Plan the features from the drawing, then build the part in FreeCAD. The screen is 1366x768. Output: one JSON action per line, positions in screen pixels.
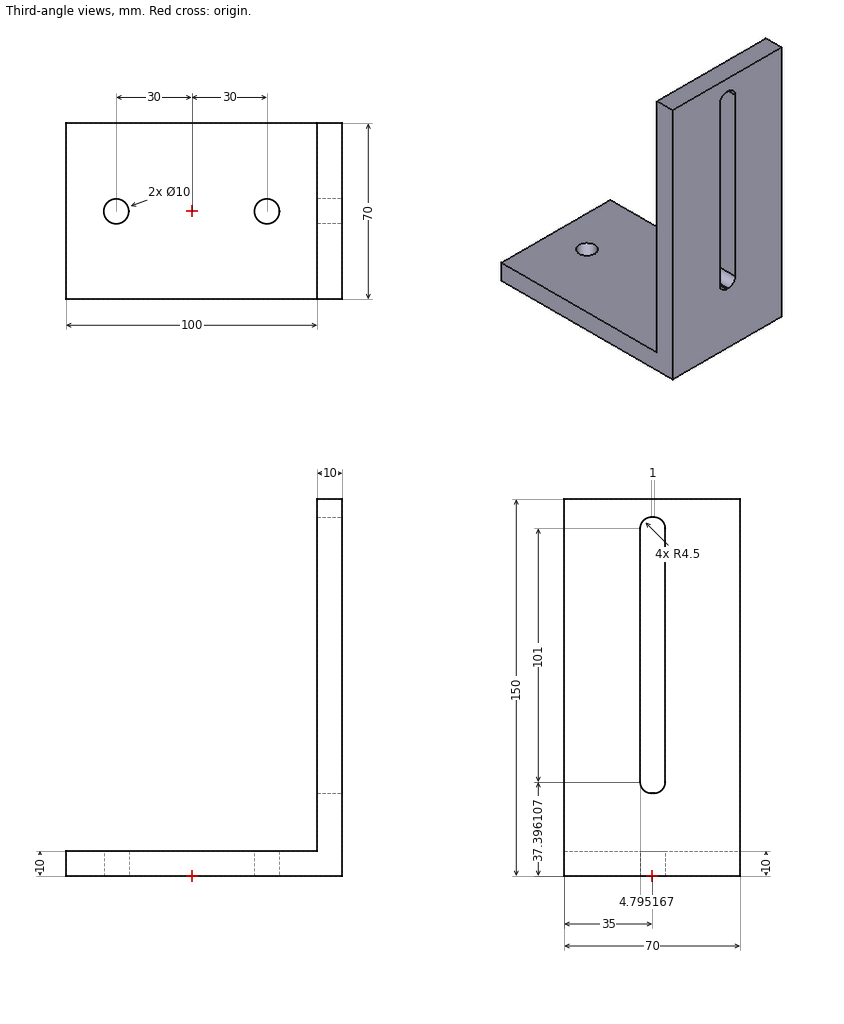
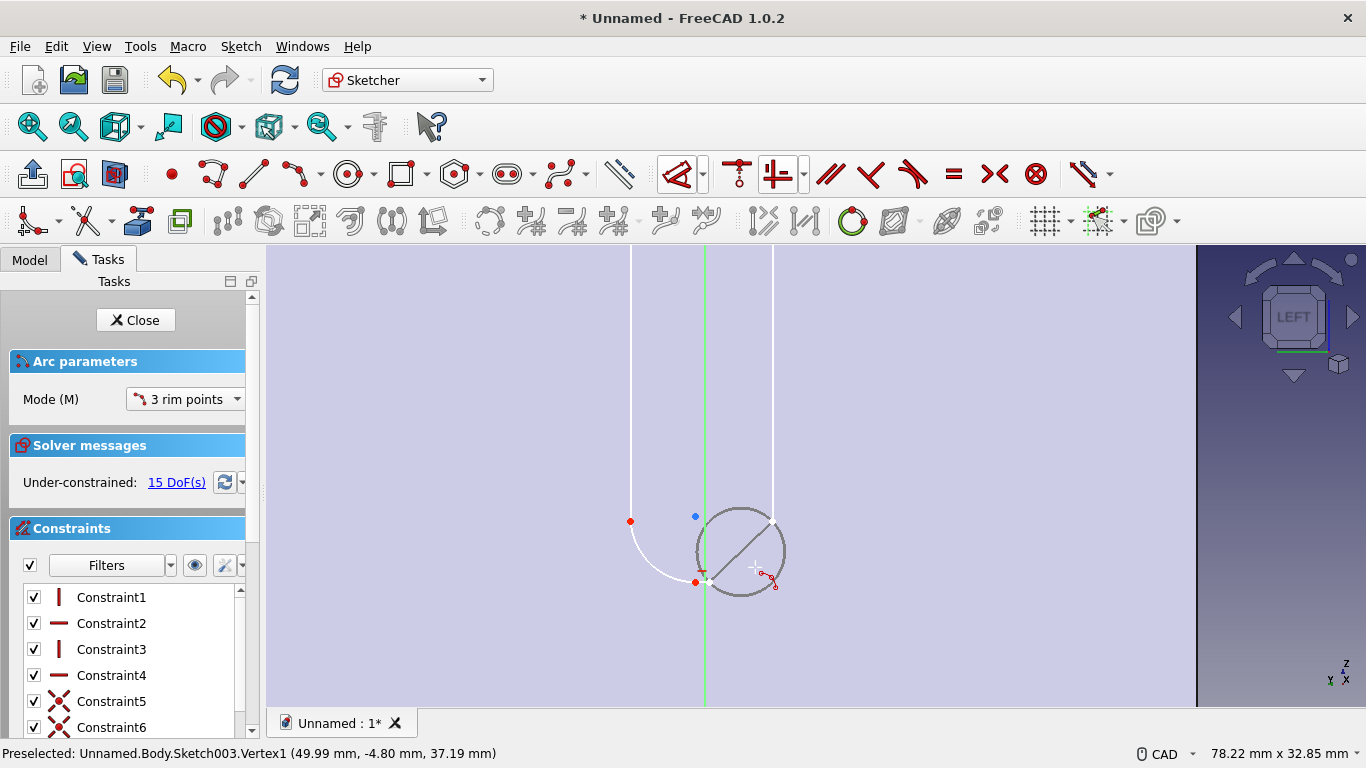
{"action": "left_click", "coordinate": [754, 563]}
{"action": "key", "text": "Escape"}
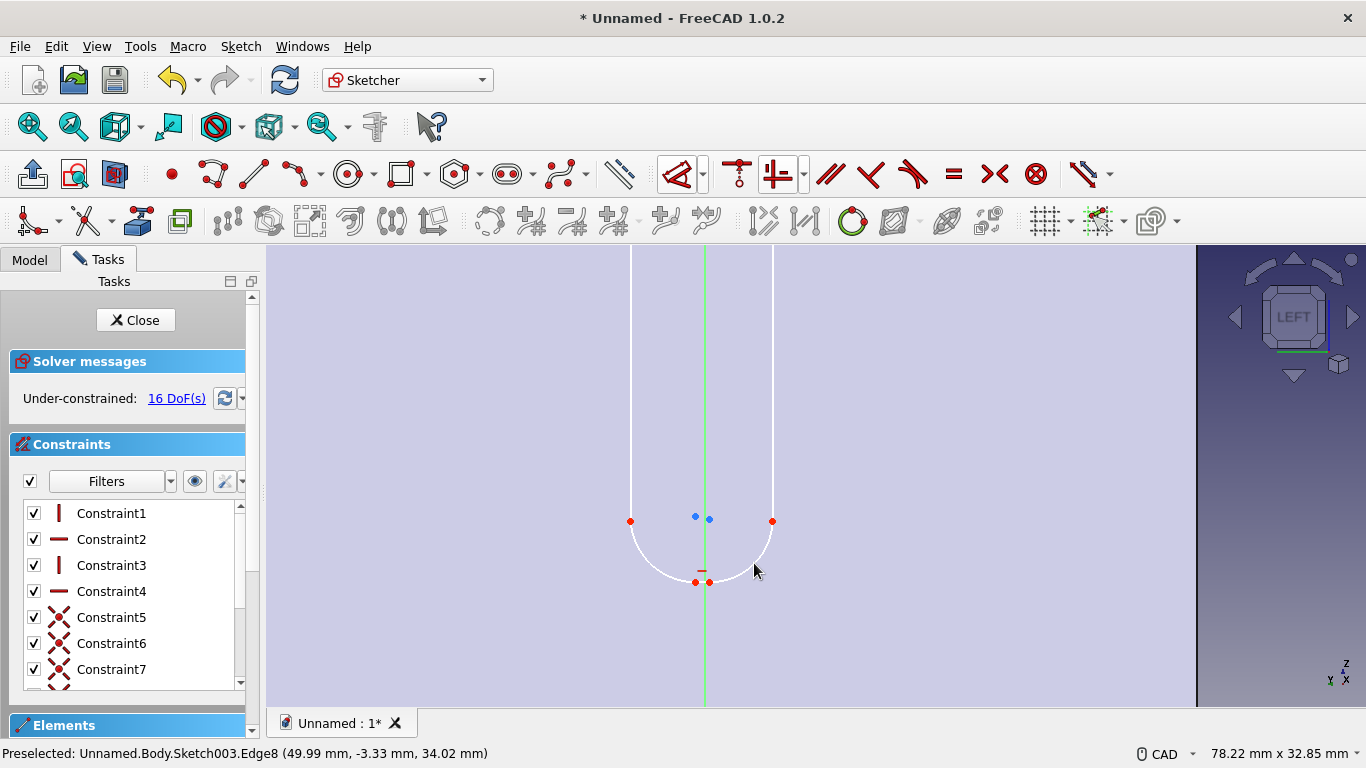
{"action": "scroll", "coordinate": [755, 544], "scroll_direction": "down", "scroll_amount": 10}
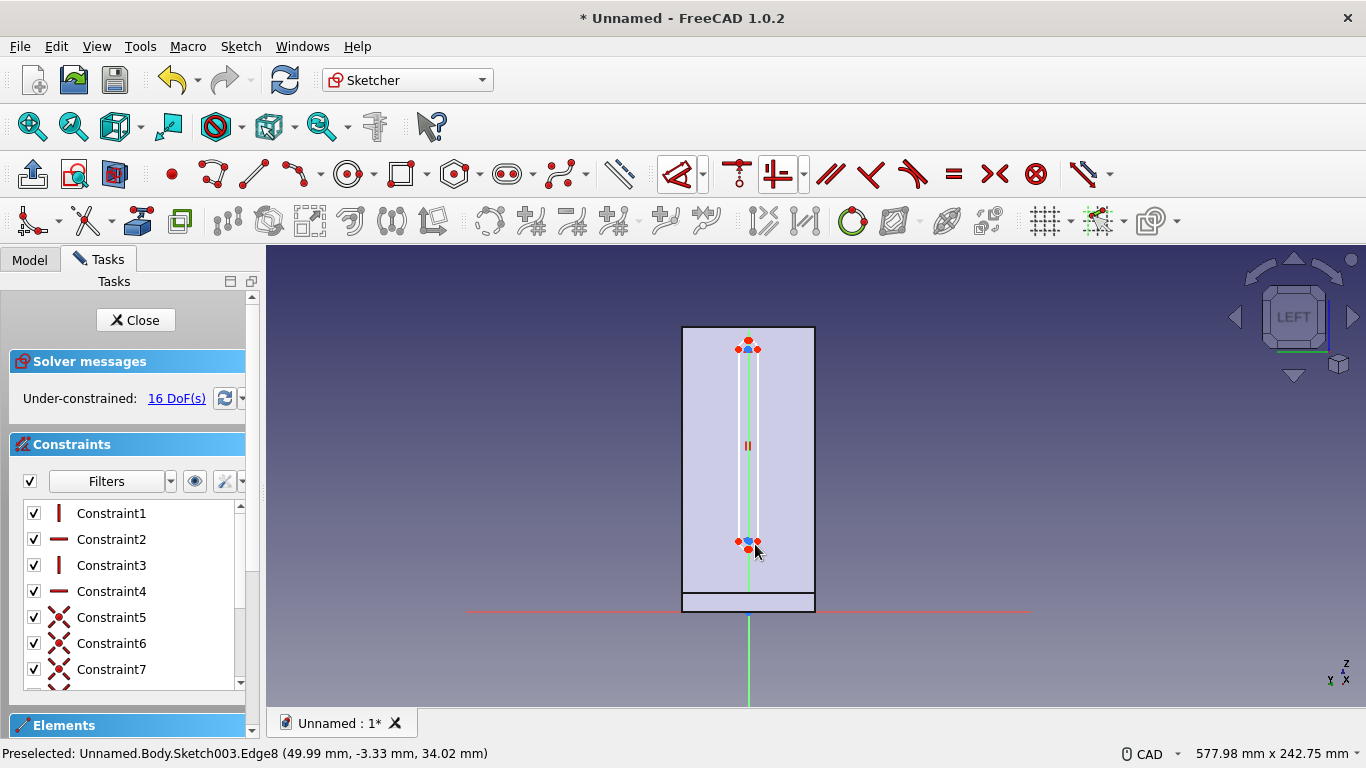
{"action": "scroll", "coordinate": [758, 484], "scroll_direction": "up", "scroll_amount": 3}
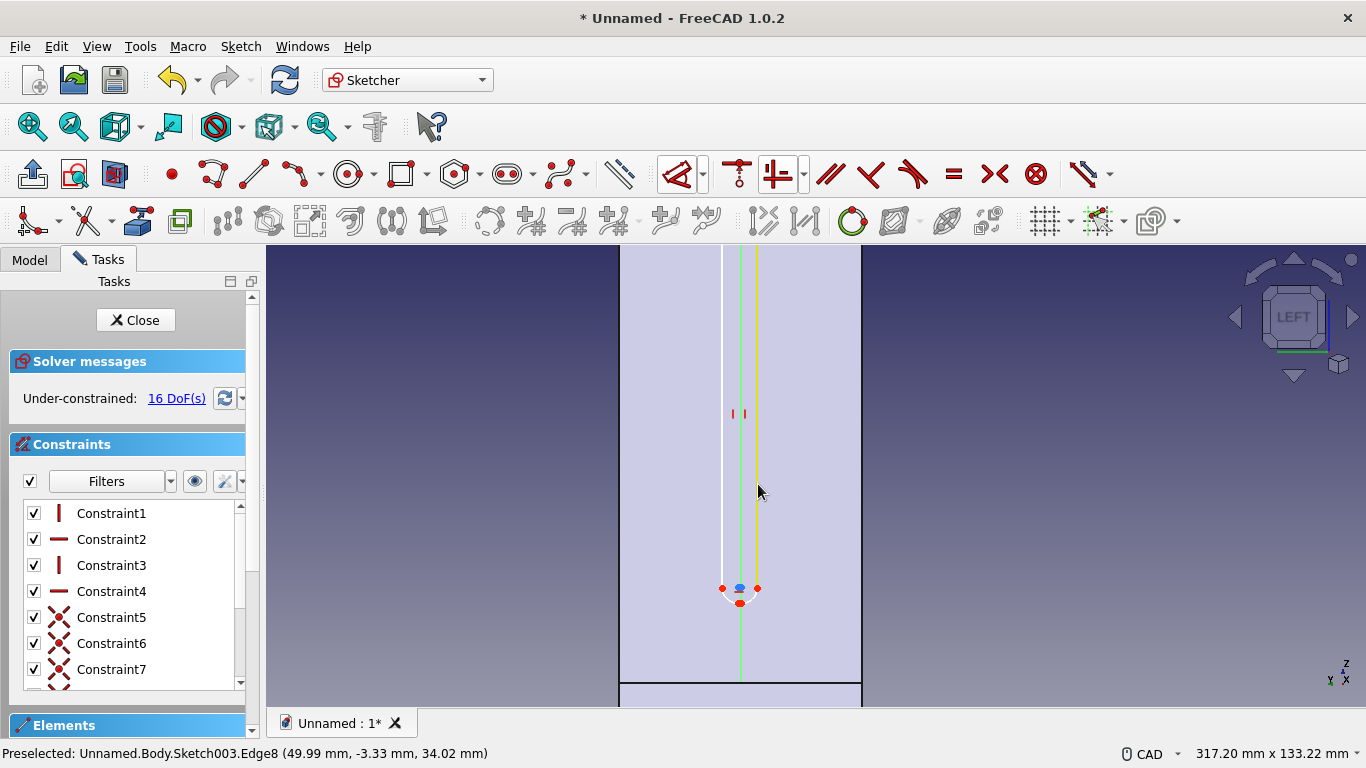
{"action": "left_click", "coordinate": [757, 483]}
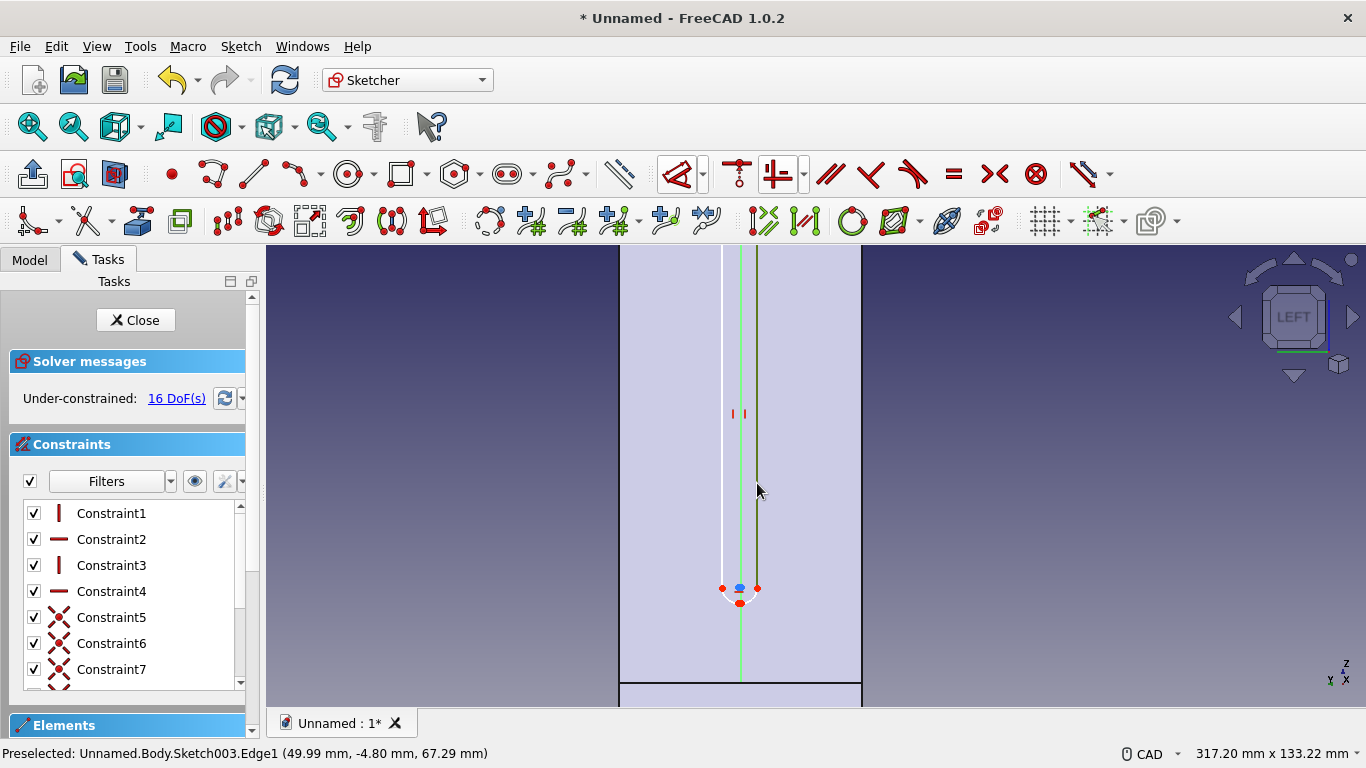
{"action": "scroll", "coordinate": [757, 484], "scroll_direction": "down", "scroll_amount": 3}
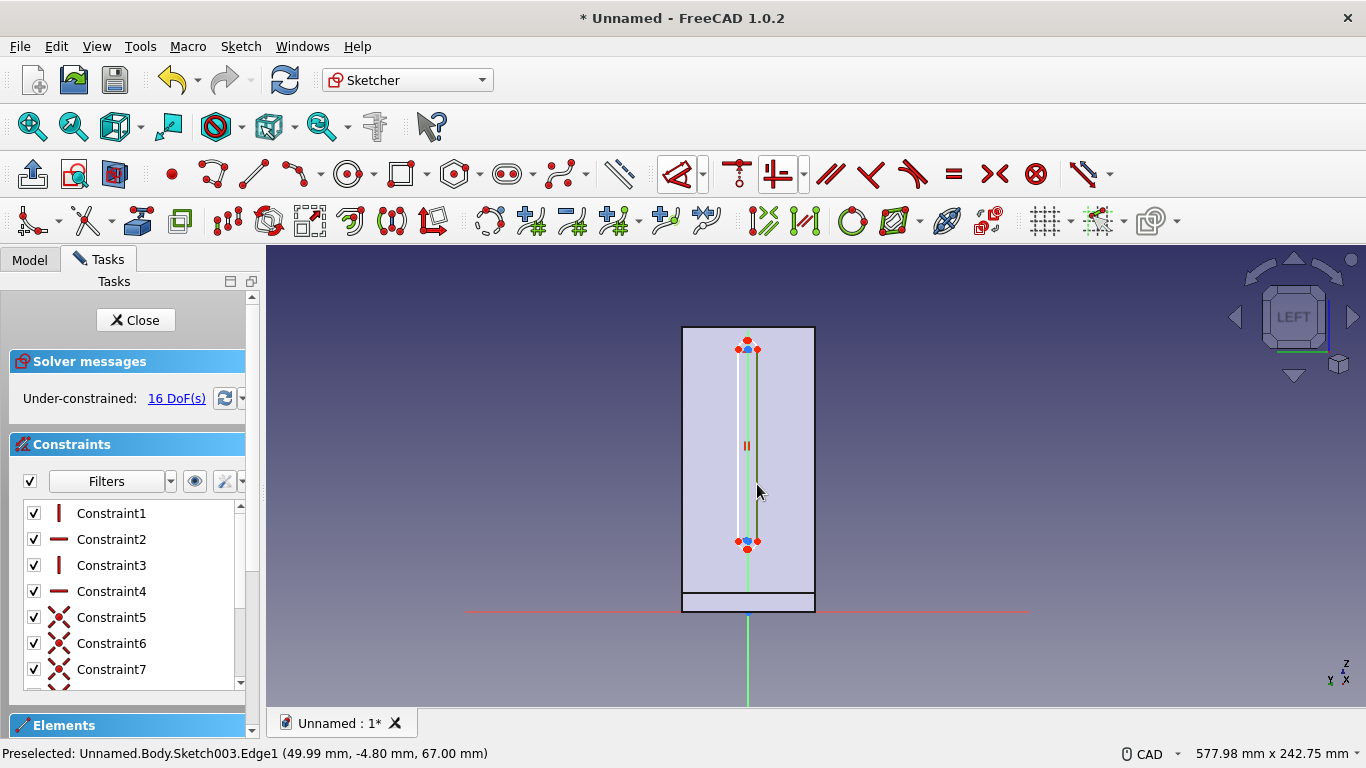
{"action": "scroll", "coordinate": [755, 343], "scroll_direction": "up", "scroll_amount": 4}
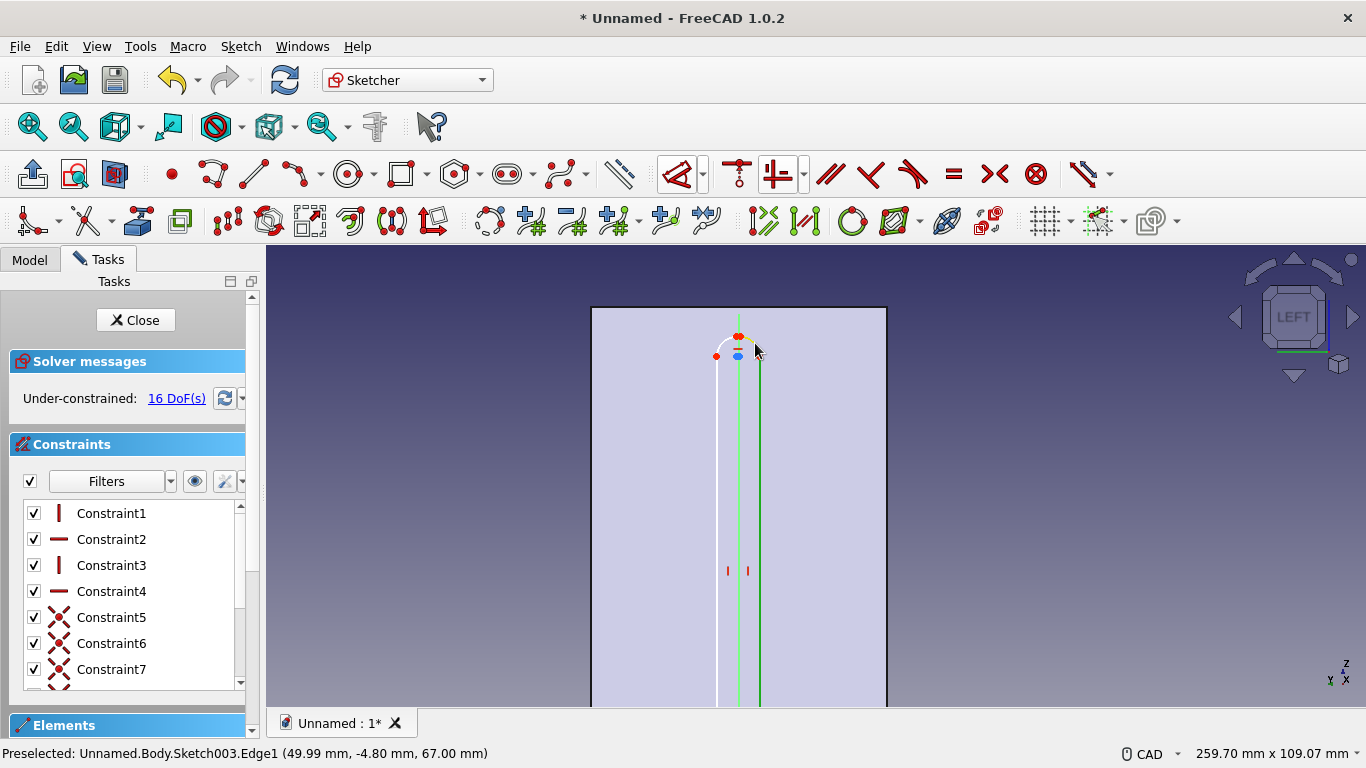
{"action": "left_click", "coordinate": [754, 343]}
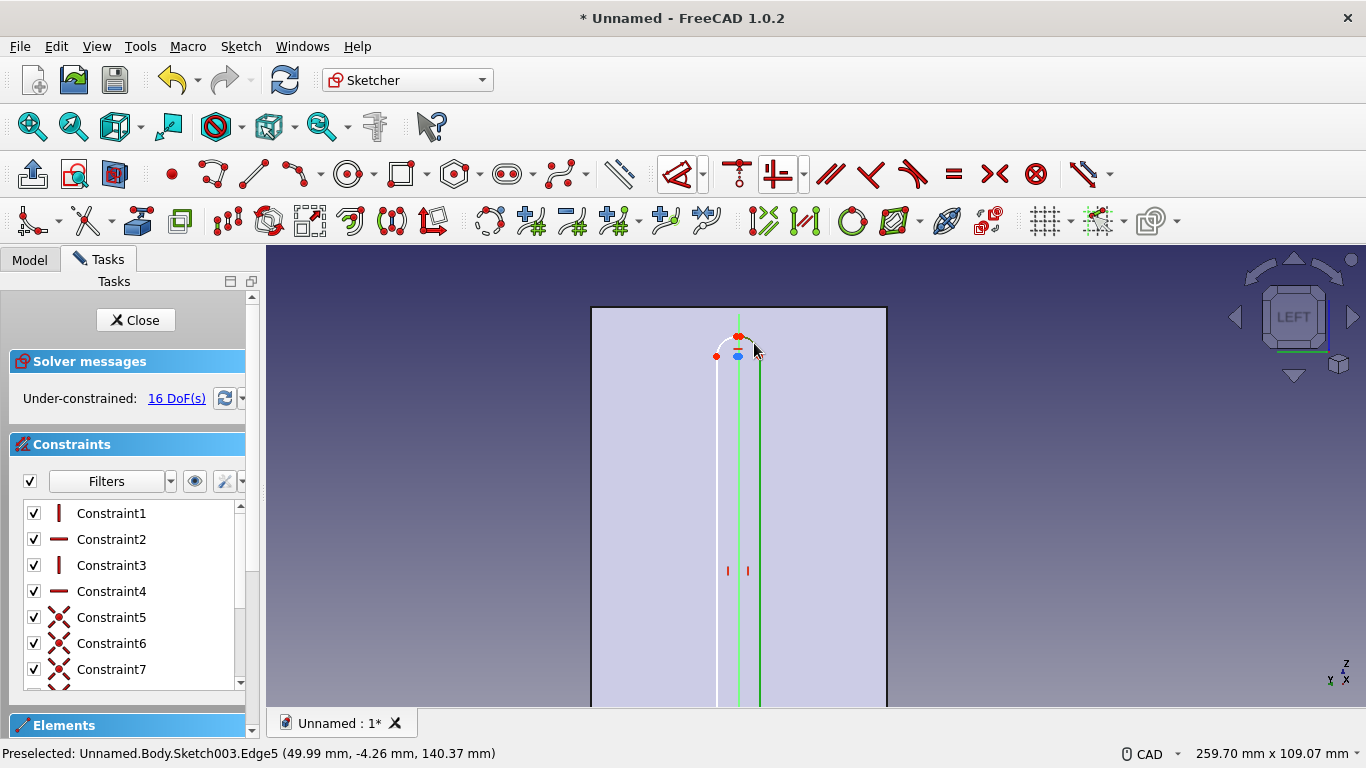
{"action": "left_click", "coordinate": [913, 174]}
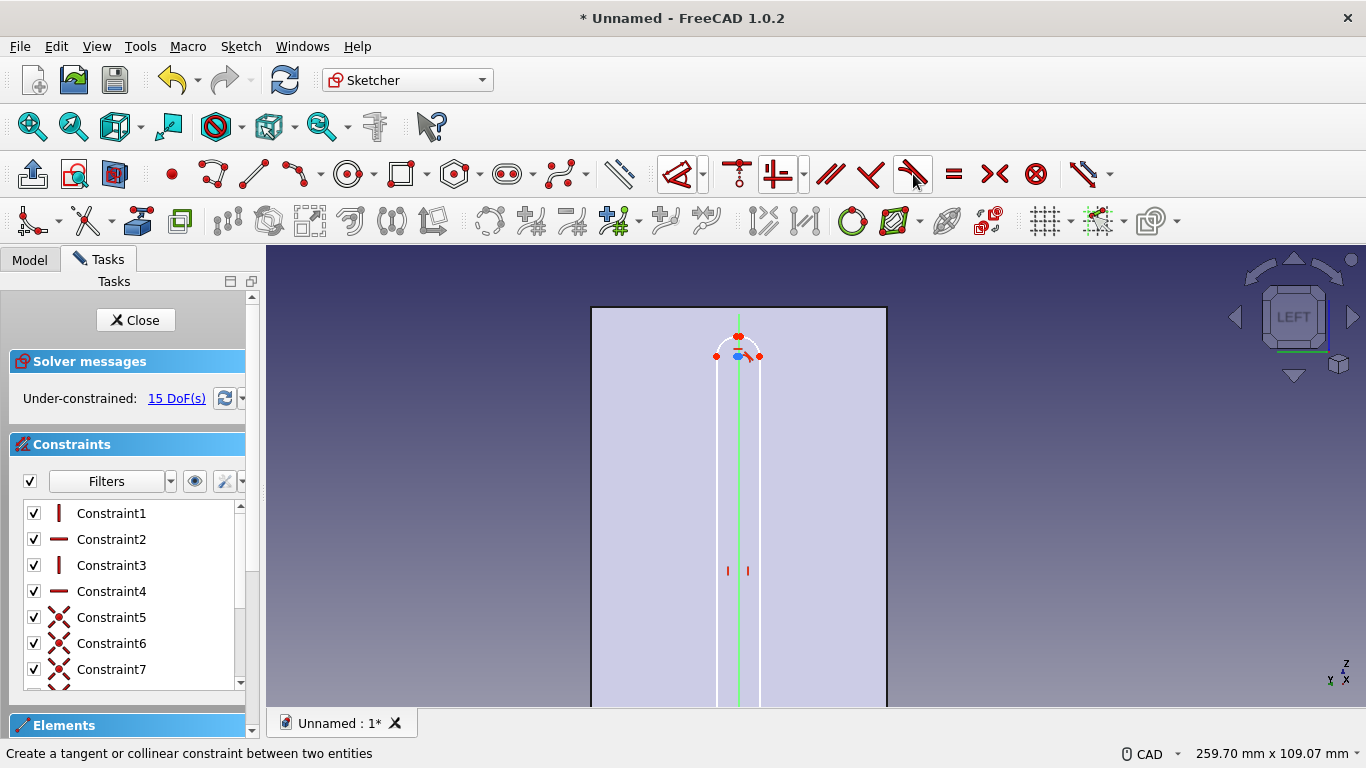
{"action": "left_click", "coordinate": [760, 656]}